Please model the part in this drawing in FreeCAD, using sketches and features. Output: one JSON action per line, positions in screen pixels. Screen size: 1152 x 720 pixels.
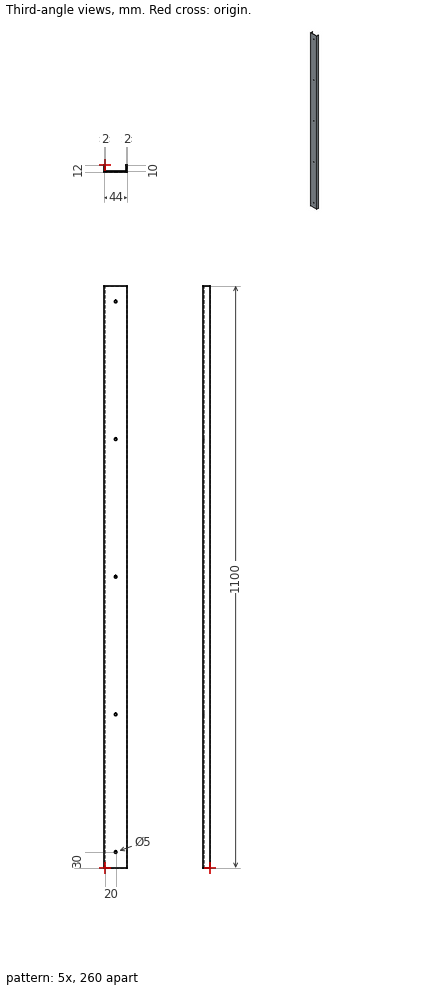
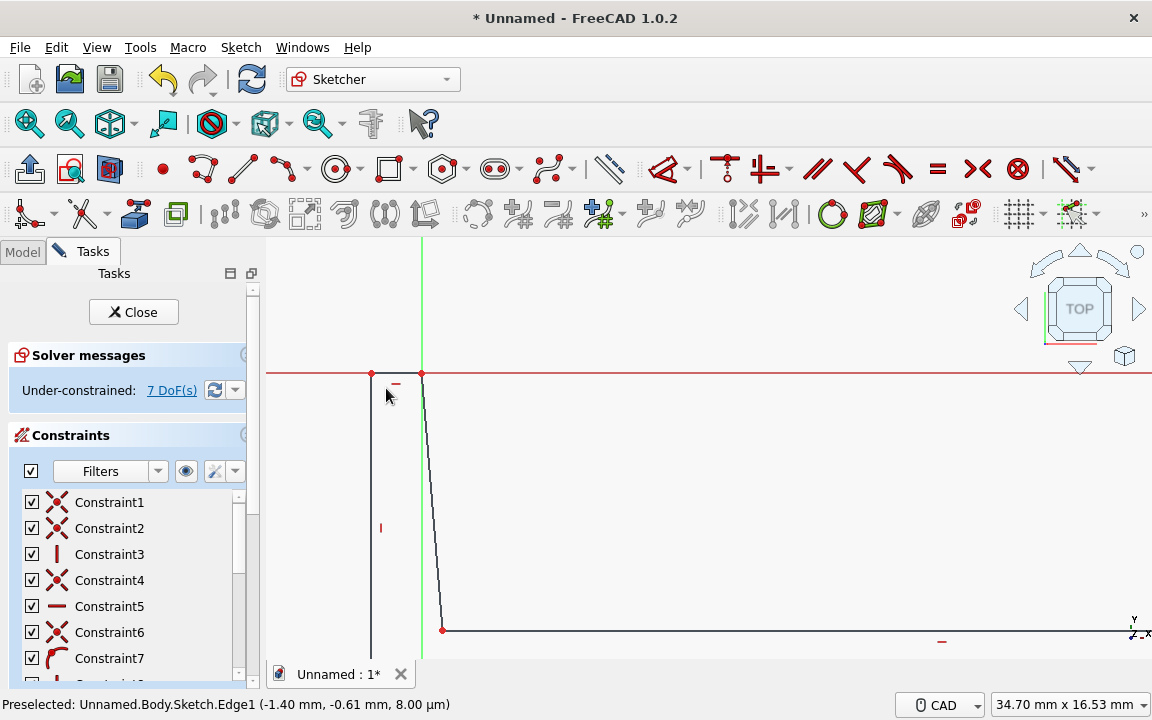
{"action": "scroll", "coordinate": [402, 384], "scroll_direction": "down", "scroll_amount": 4}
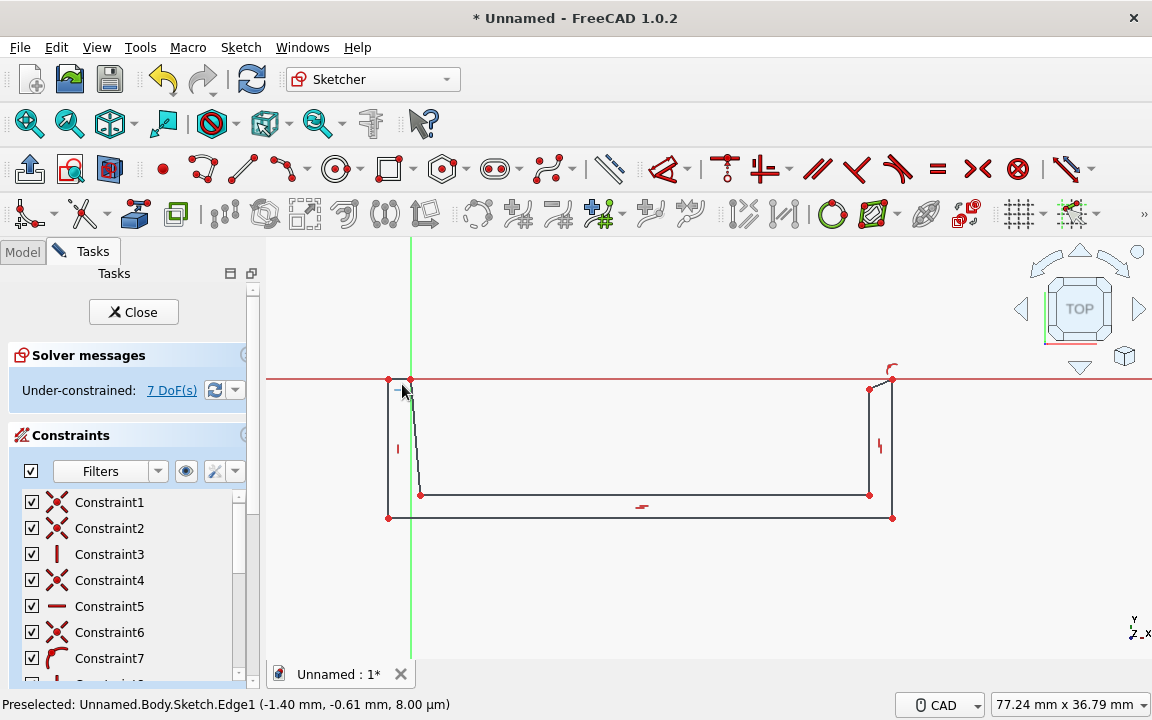
{"action": "scroll", "coordinate": [876, 386], "scroll_direction": "up", "scroll_amount": 4}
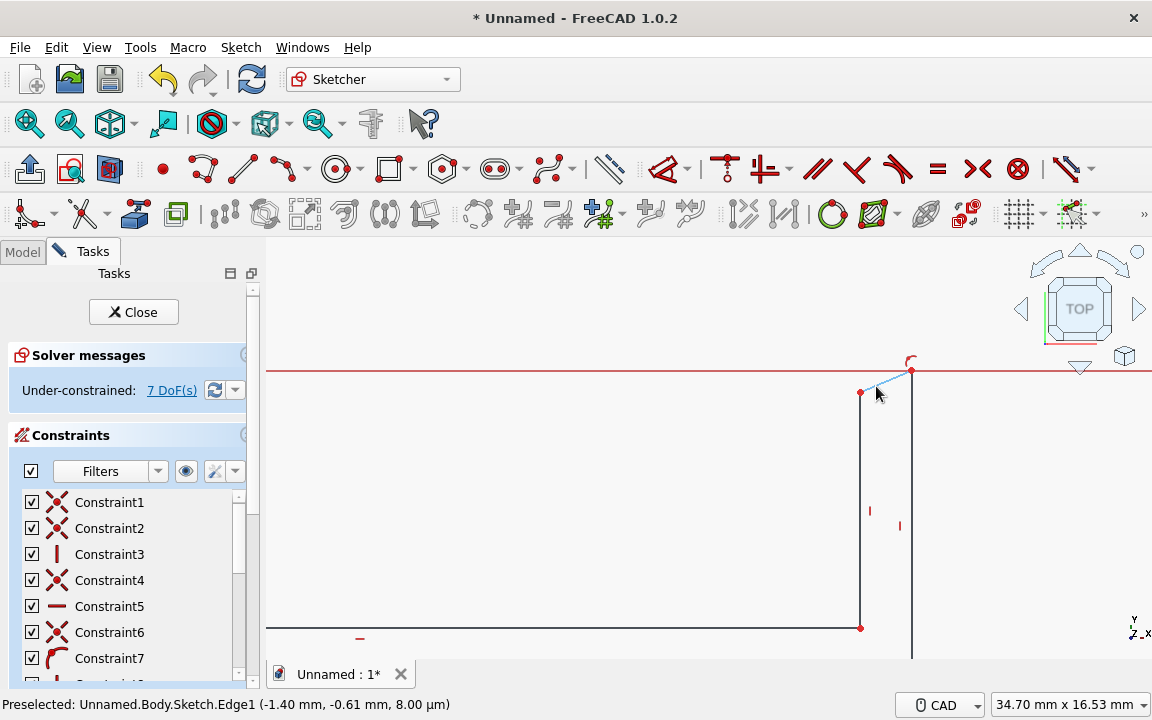
{"action": "left_click", "coordinate": [876, 386]}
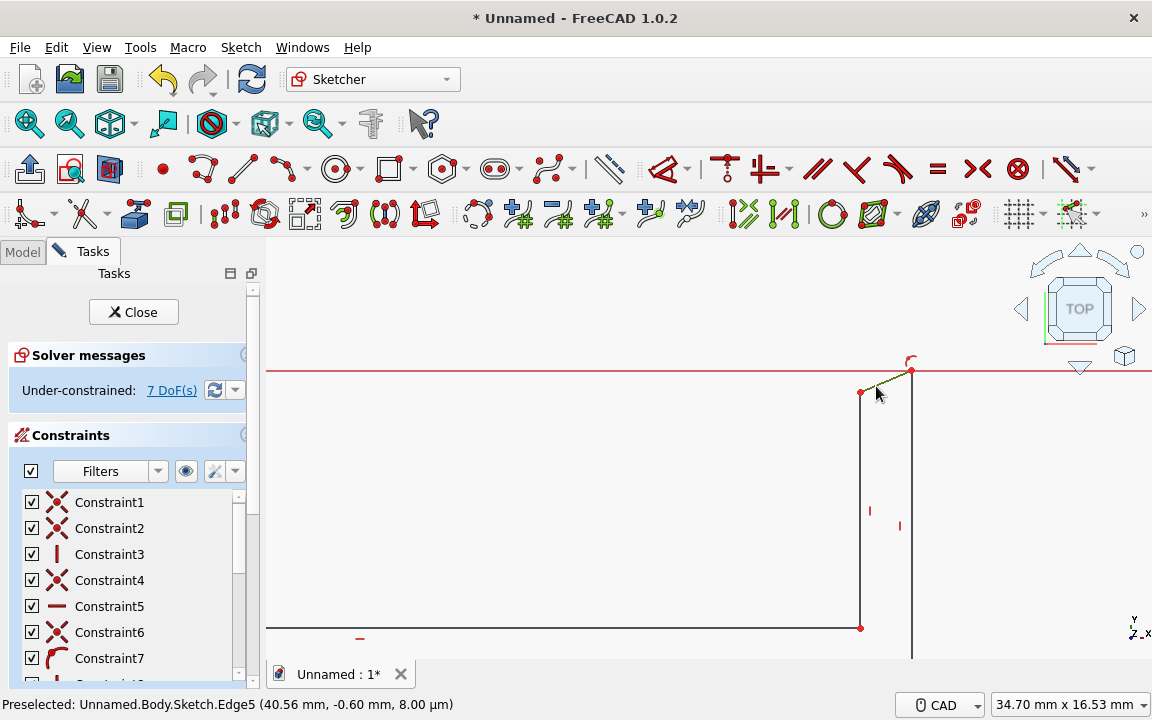
{"action": "left_click", "coordinate": [792, 170]}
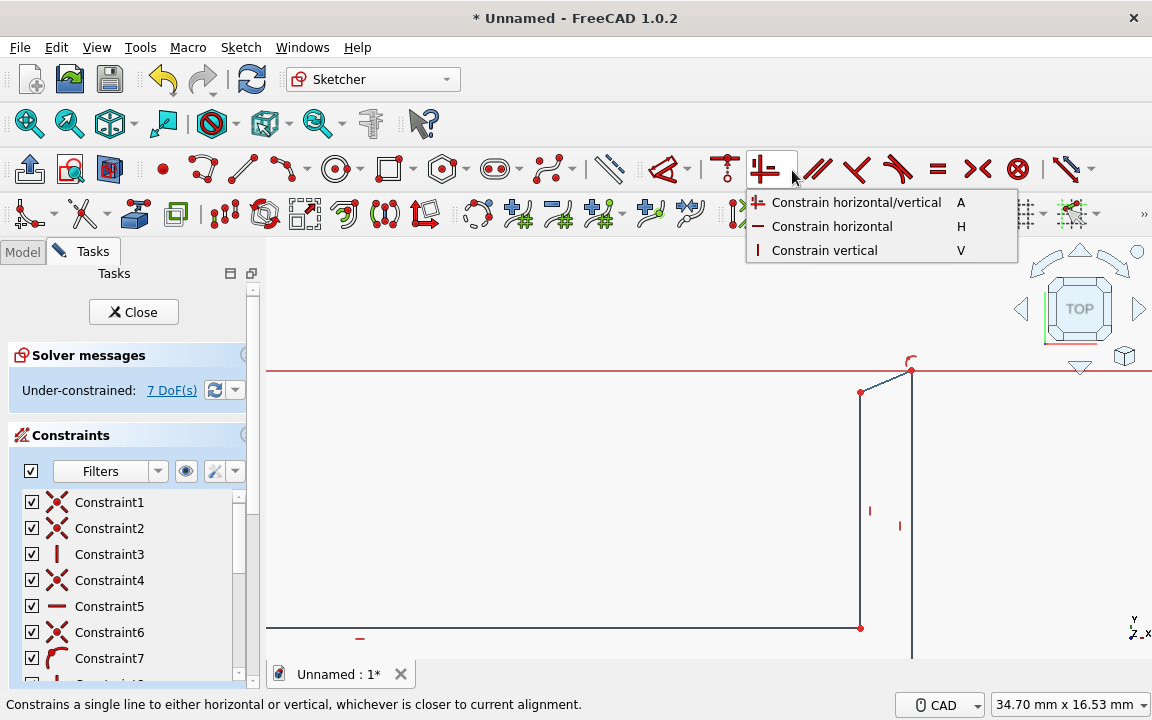
{"action": "left_click", "coordinate": [882, 226]}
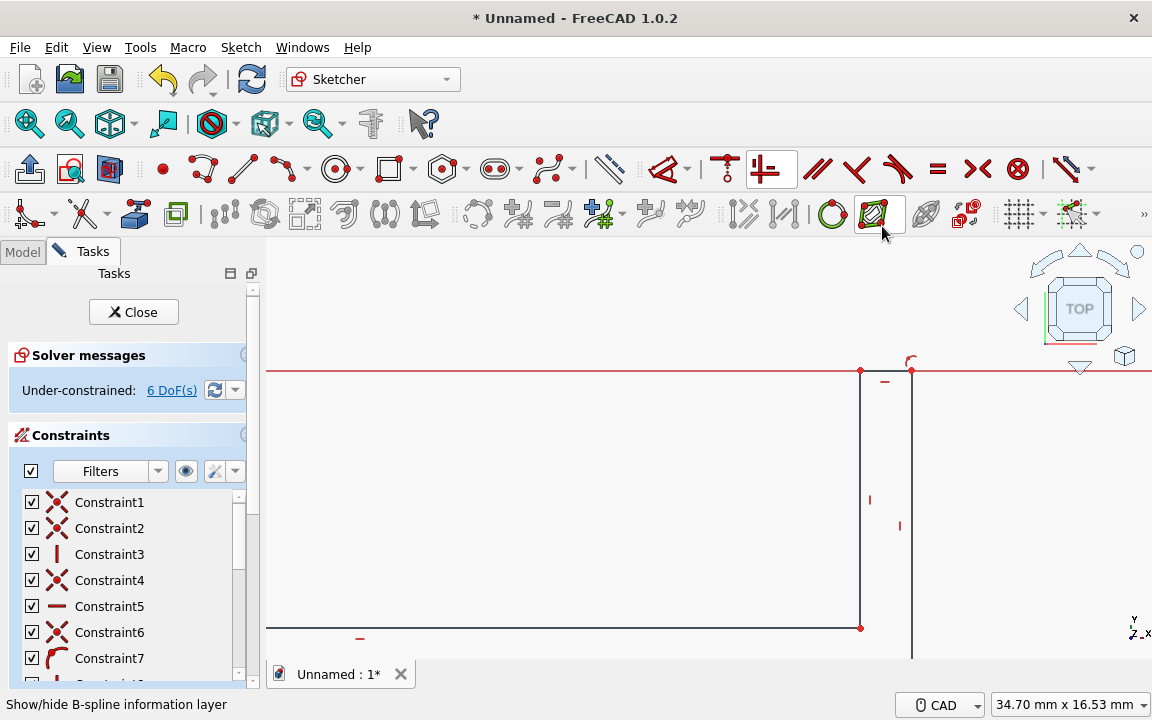
{"action": "scroll", "coordinate": [877, 386], "scroll_direction": "down", "scroll_amount": 4}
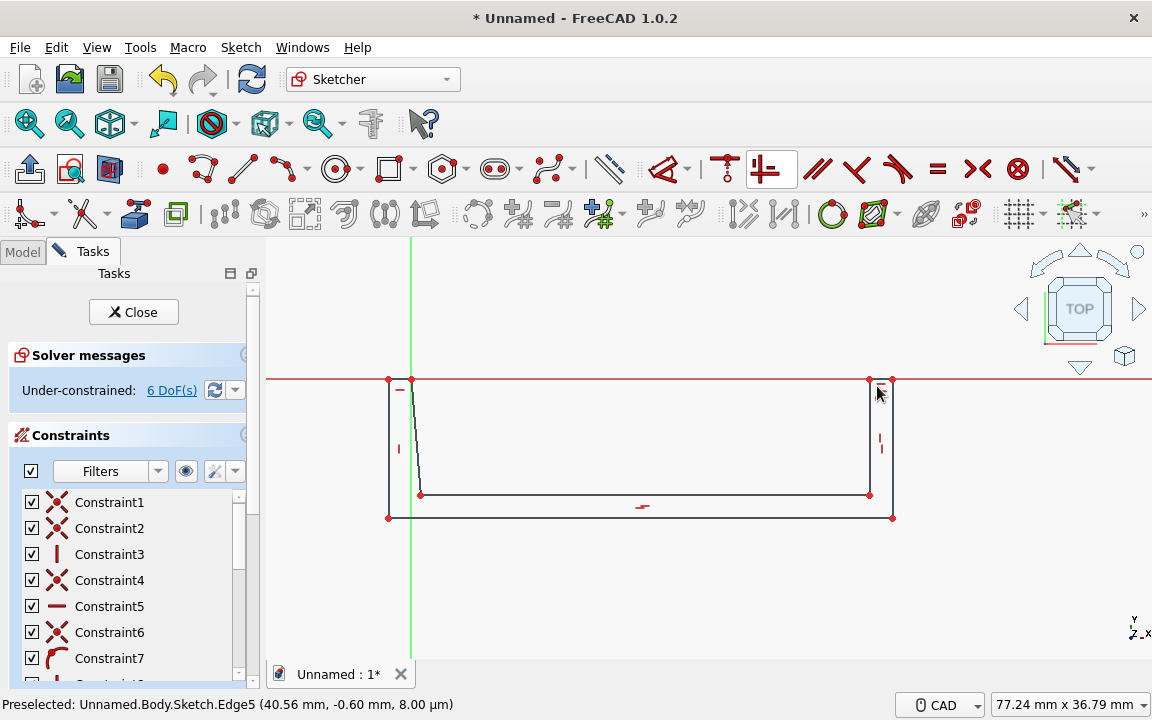
{"action": "scroll", "coordinate": [418, 460], "scroll_direction": "up", "scroll_amount": 4}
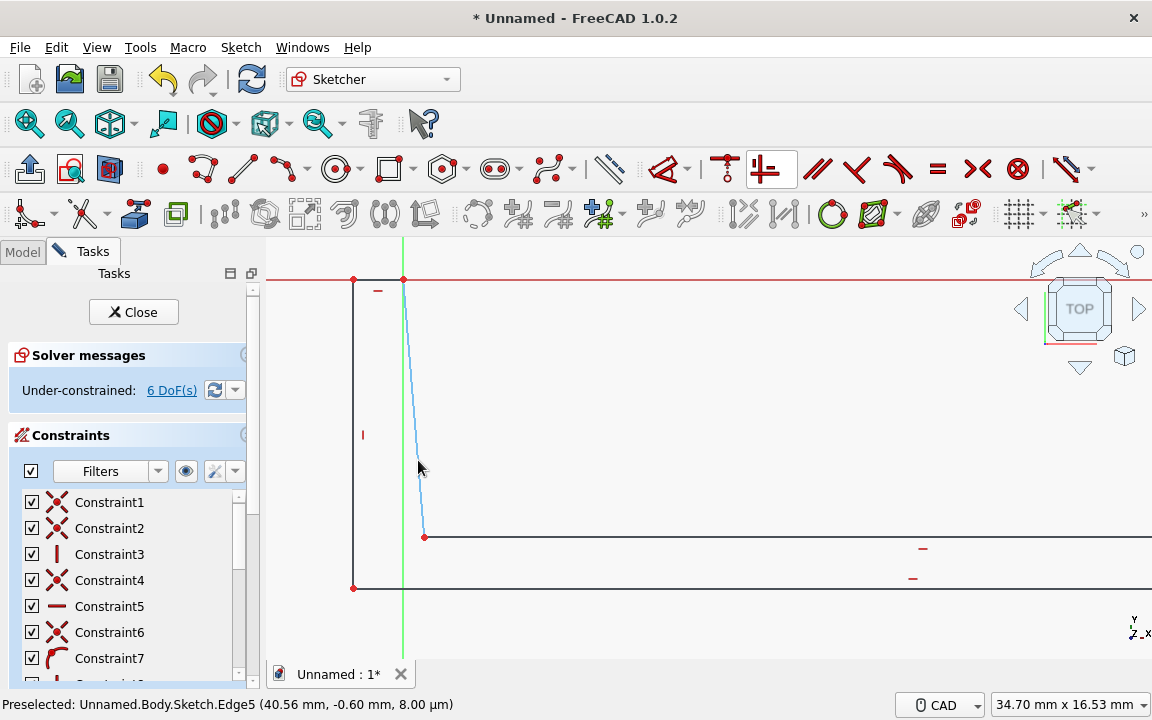
{"action": "left_click", "coordinate": [418, 460]}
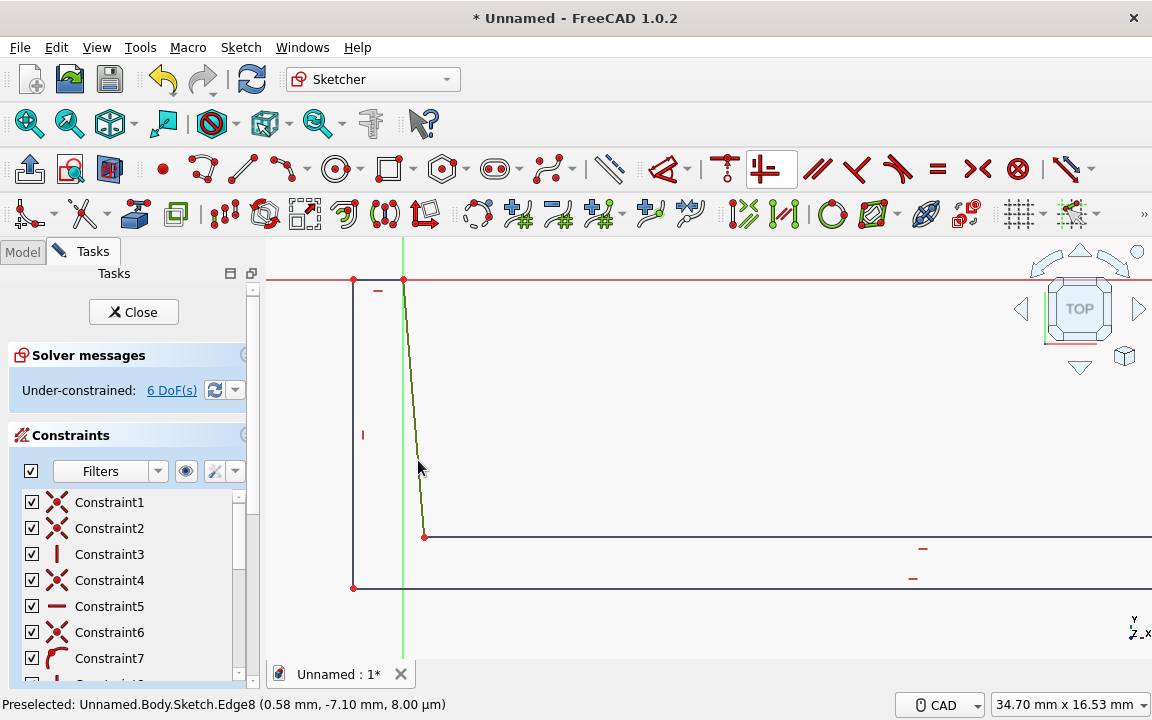
{"action": "key", "text": "v"}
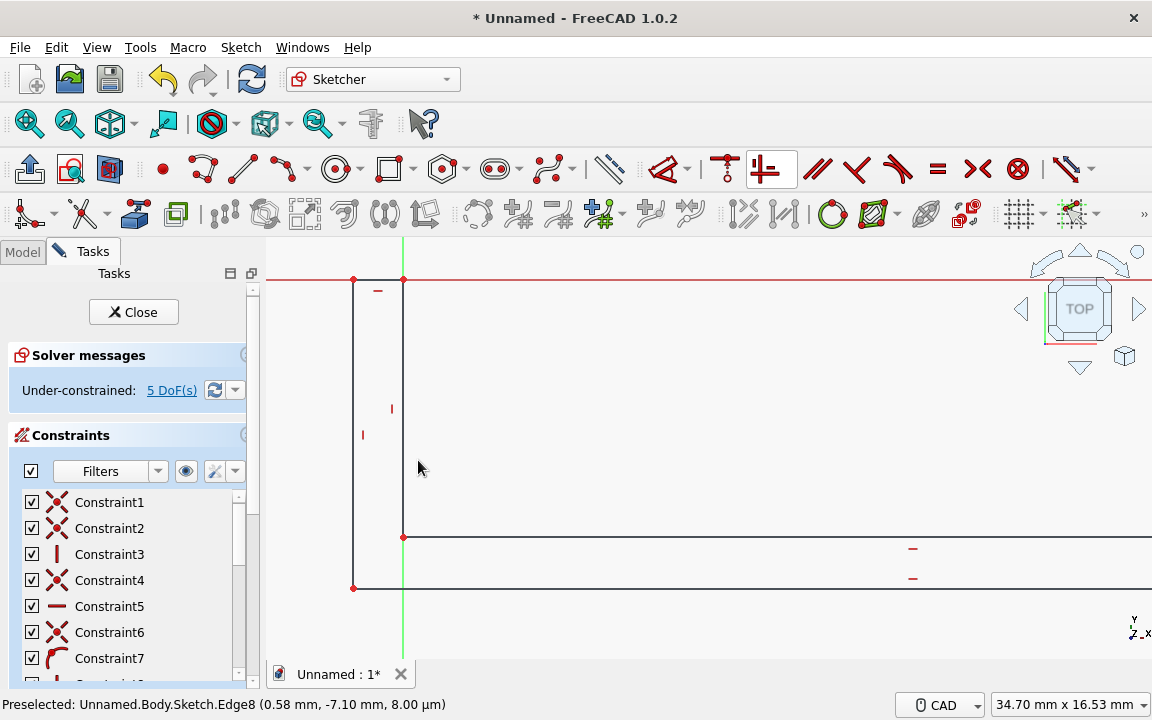
{"action": "left_click", "coordinate": [388, 280]}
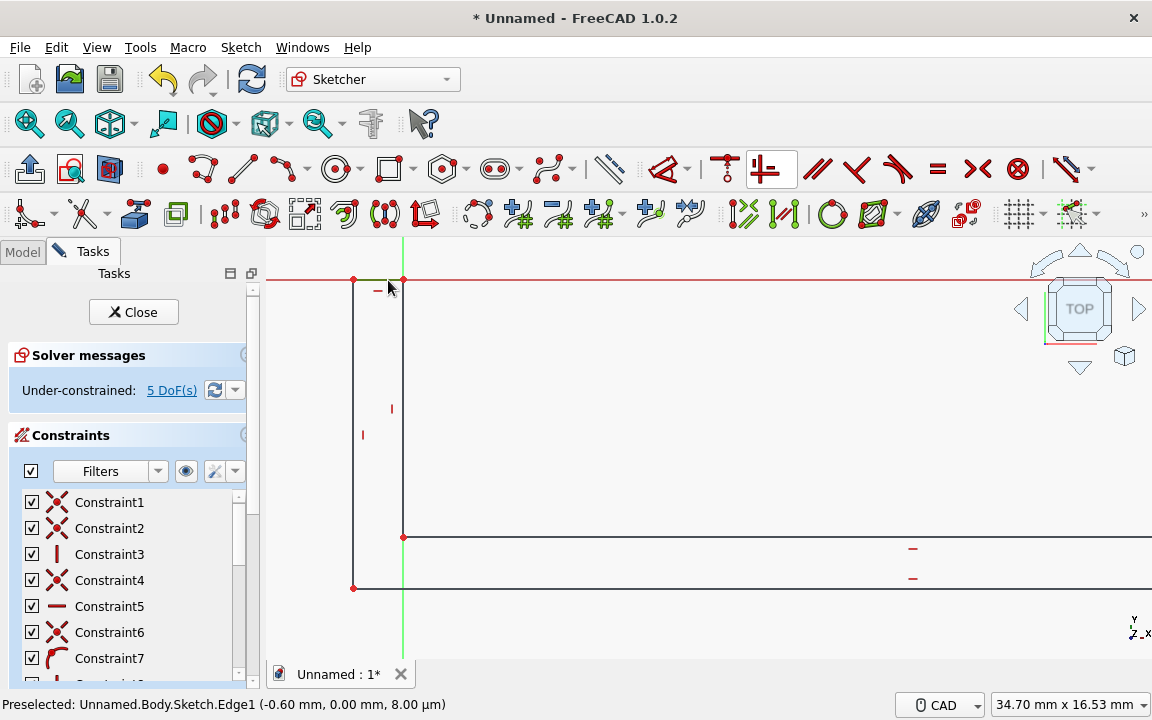
{"action": "left_click", "coordinate": [690, 170]}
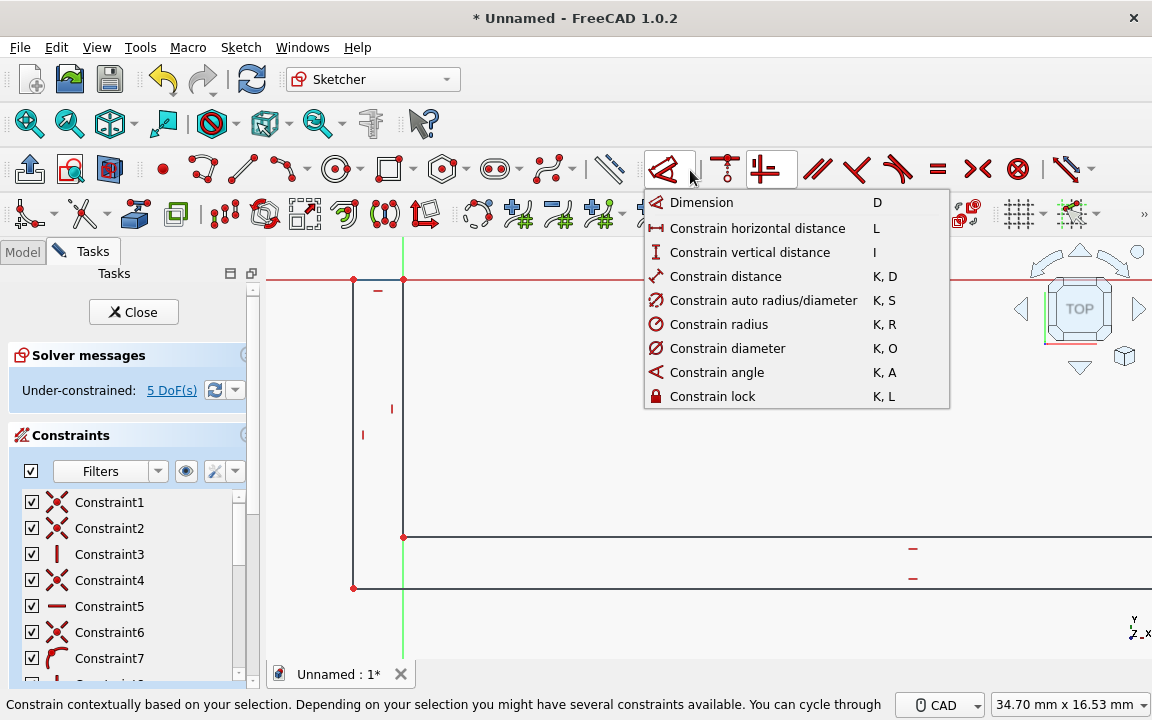
{"action": "left_click", "coordinate": [797, 228]}